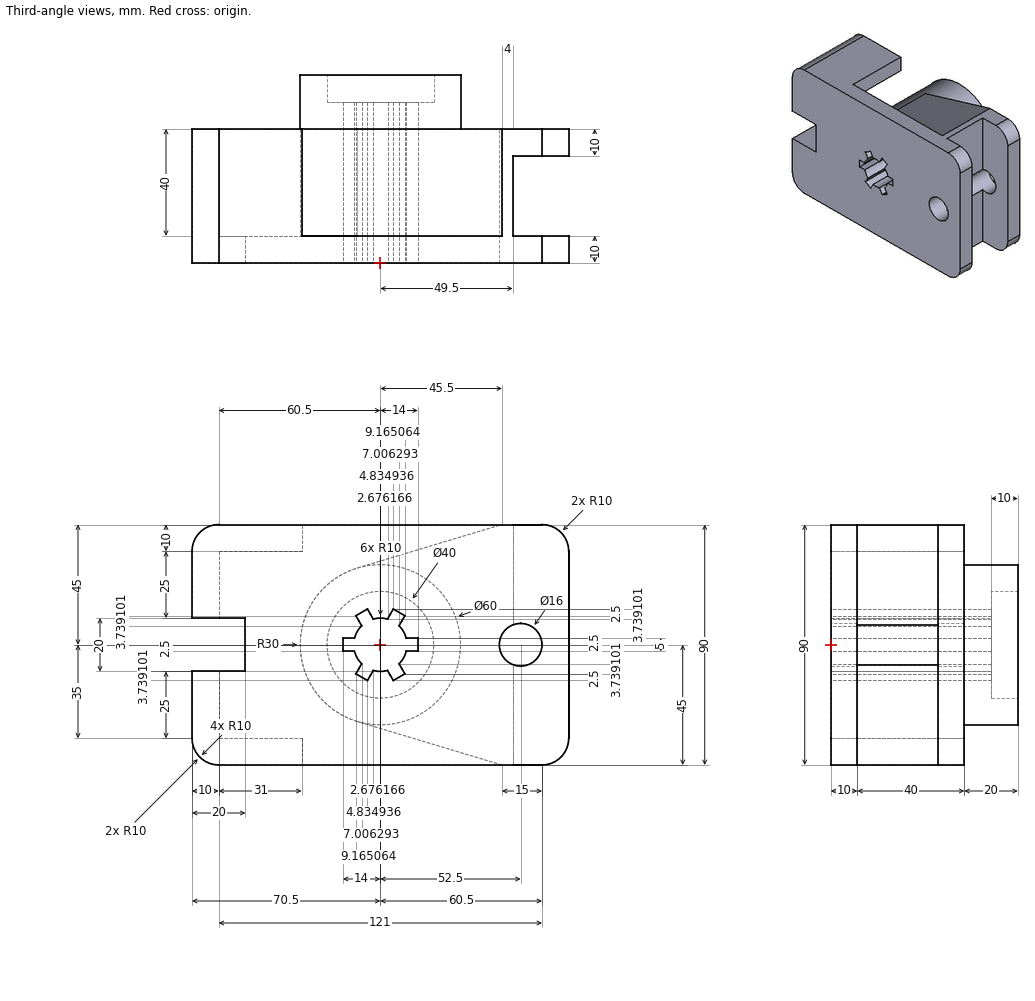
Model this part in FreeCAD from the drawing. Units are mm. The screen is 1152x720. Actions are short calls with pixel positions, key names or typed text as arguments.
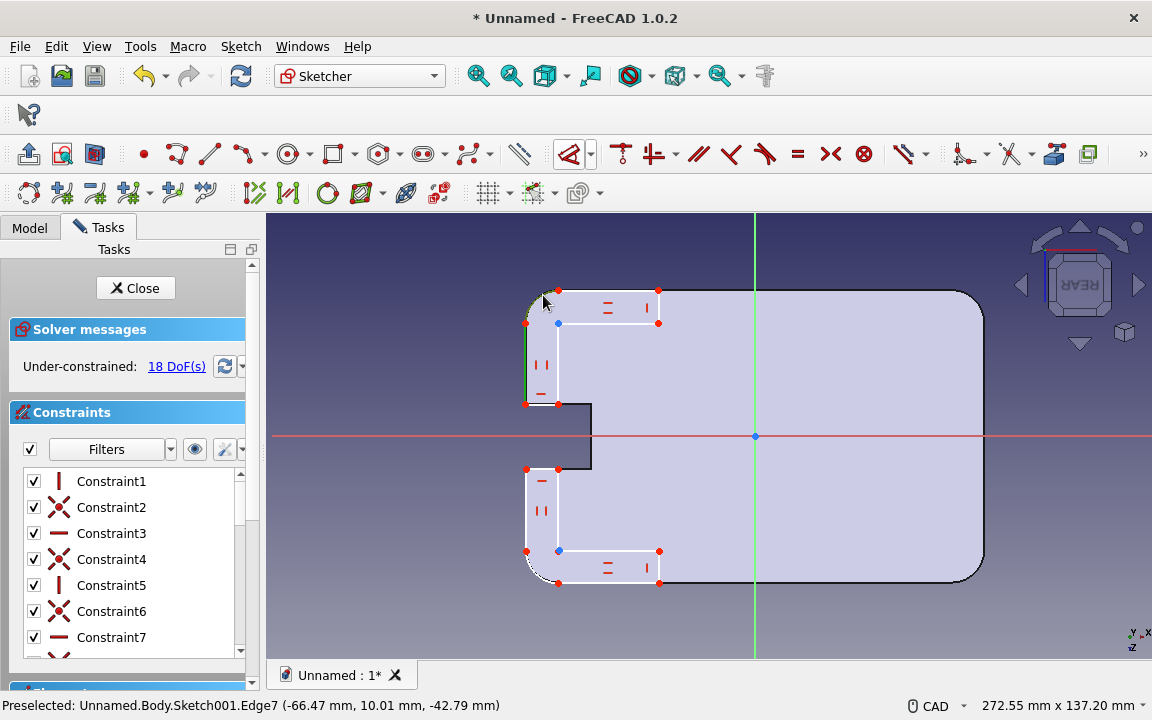
click(765, 154)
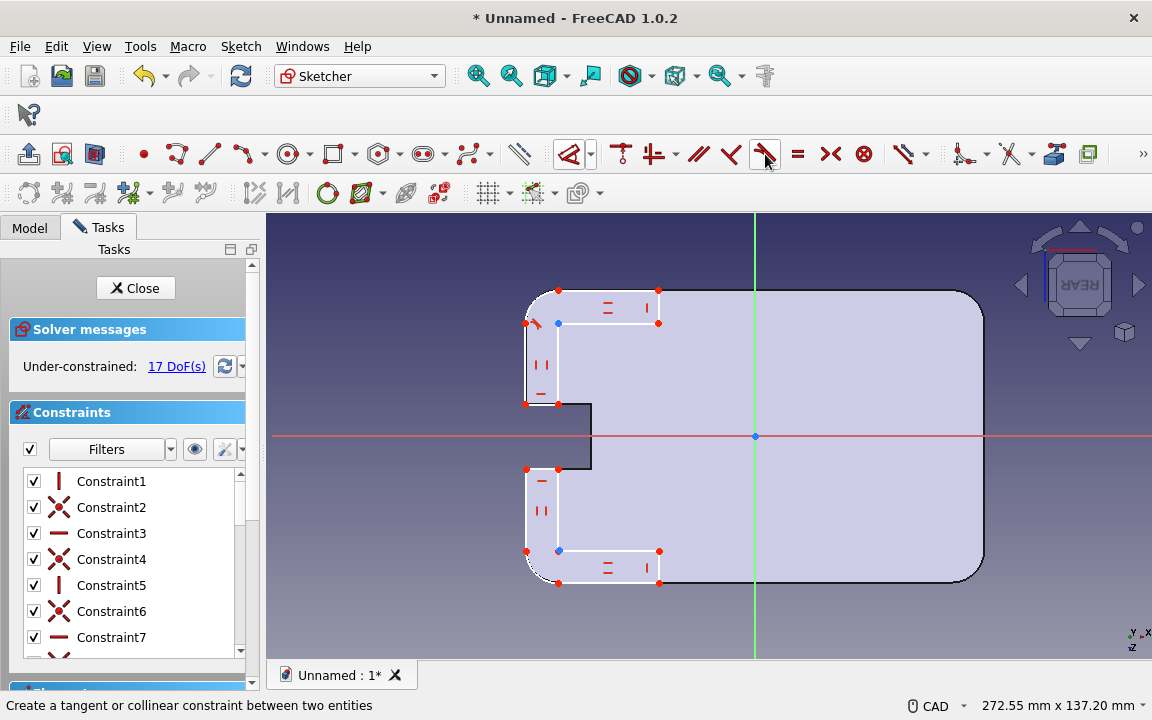
click(629, 291)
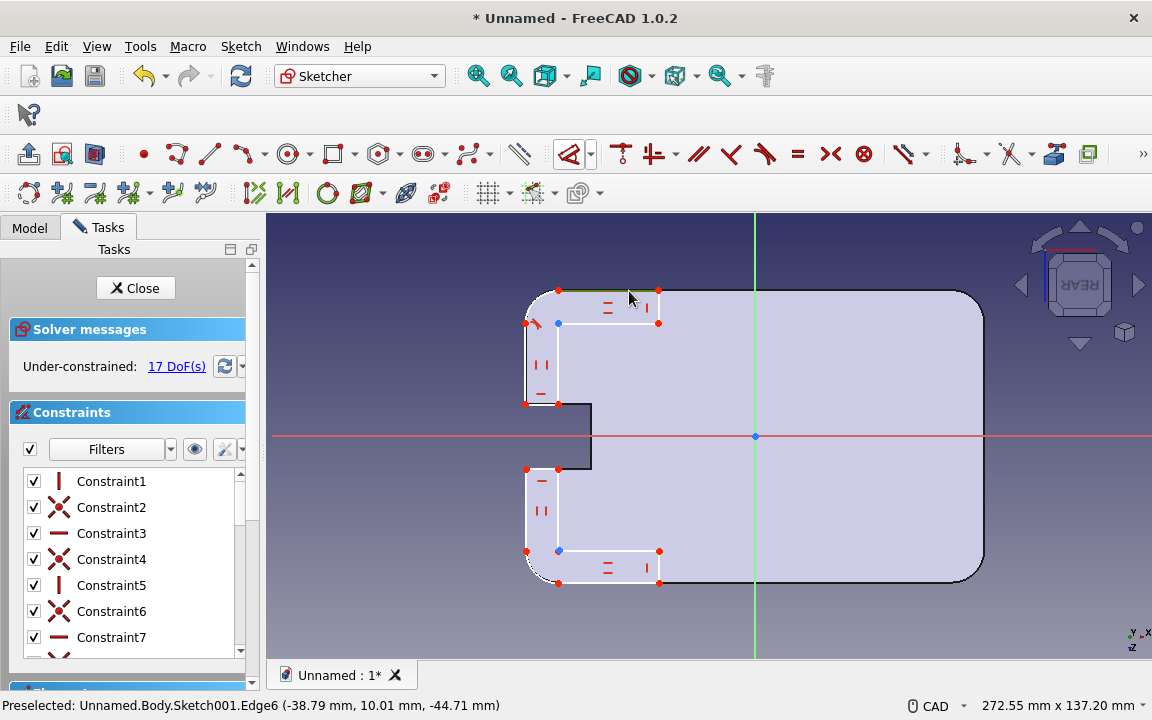
click(543, 295)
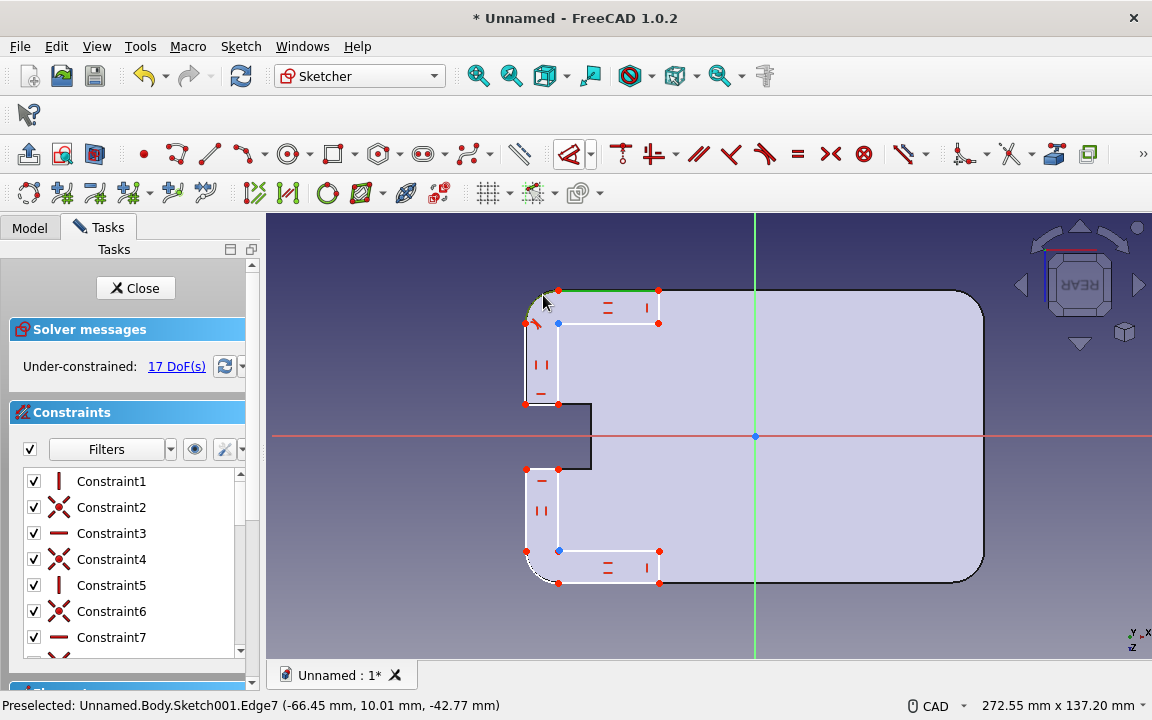
click(765, 154)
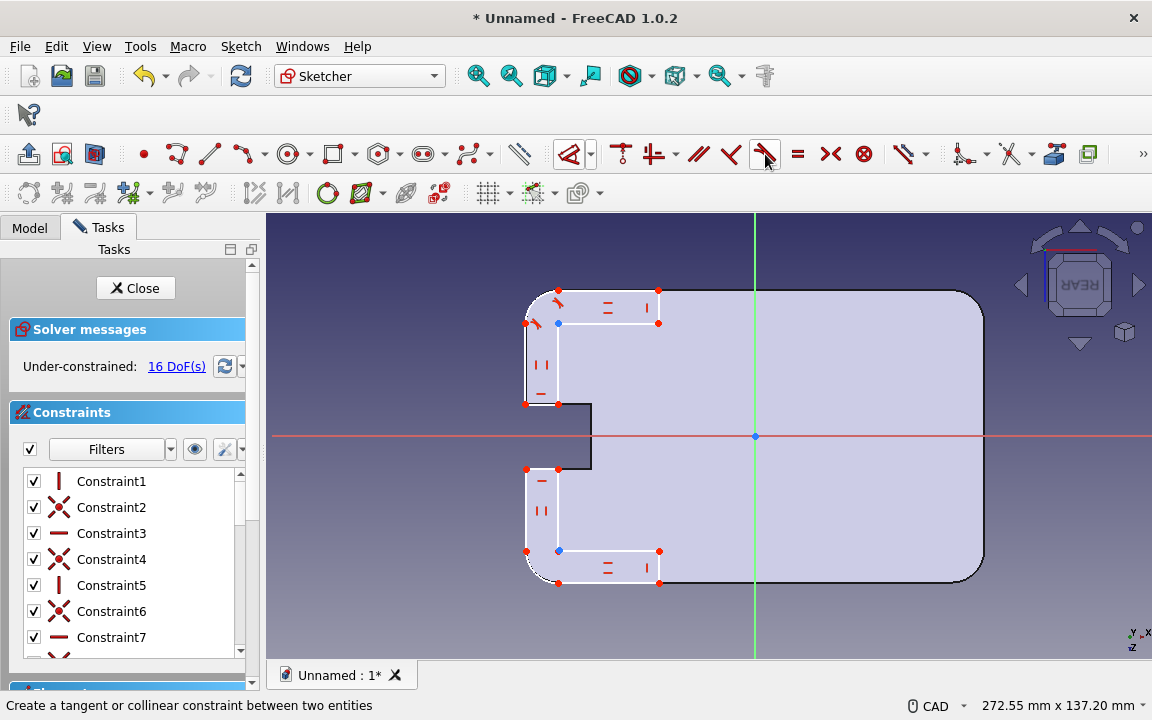
click(588, 583)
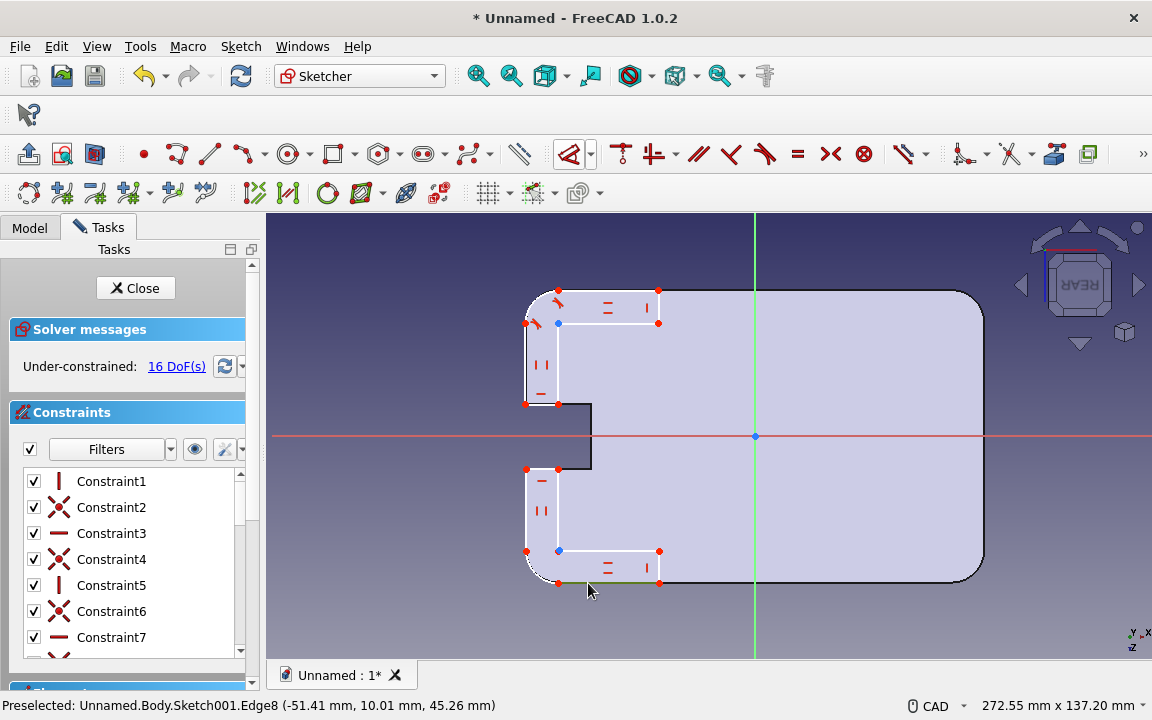
click(530, 566)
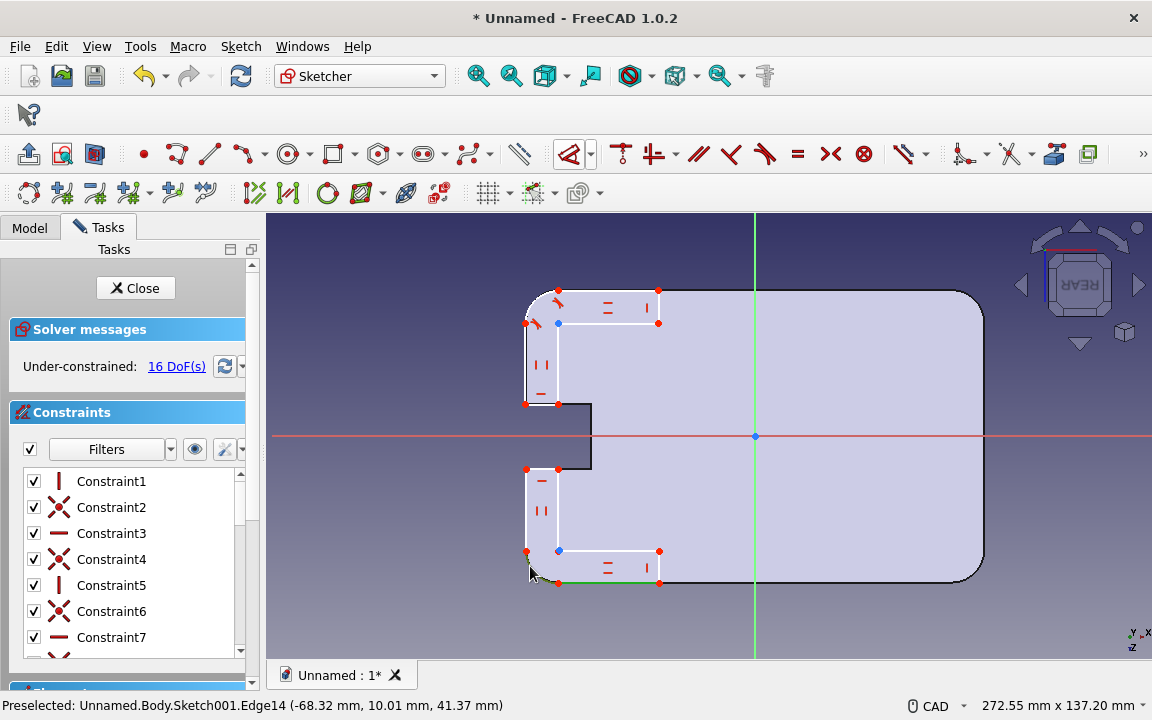
click(765, 154)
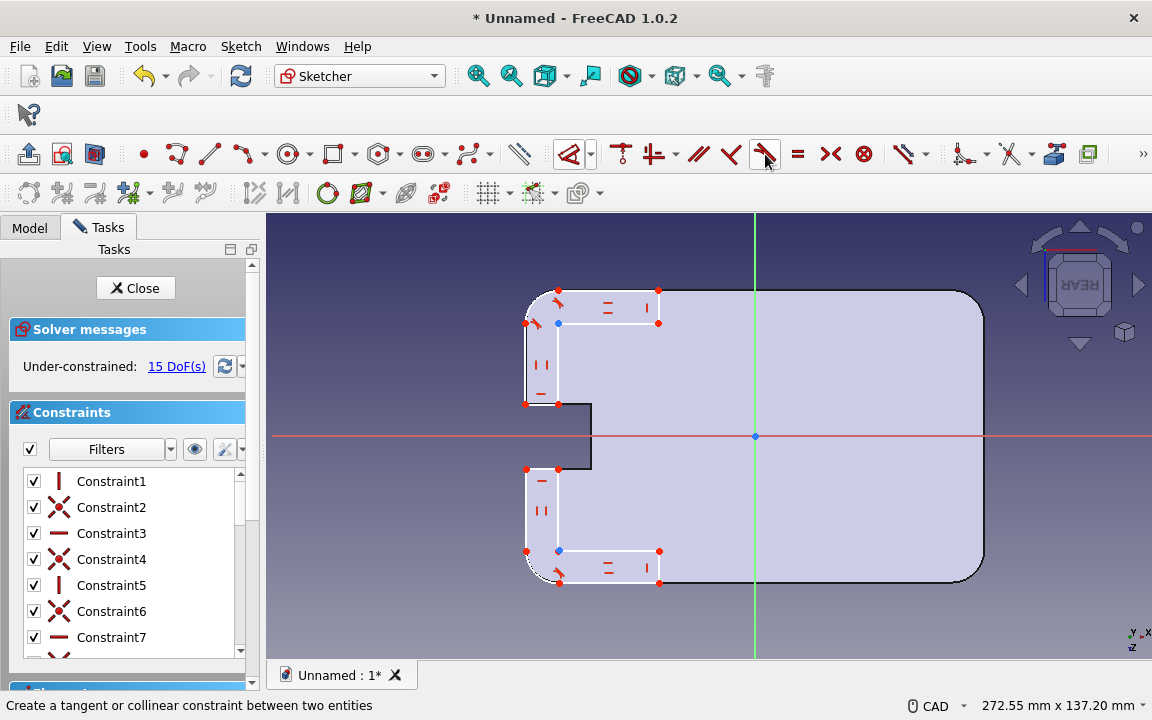
click(526, 494)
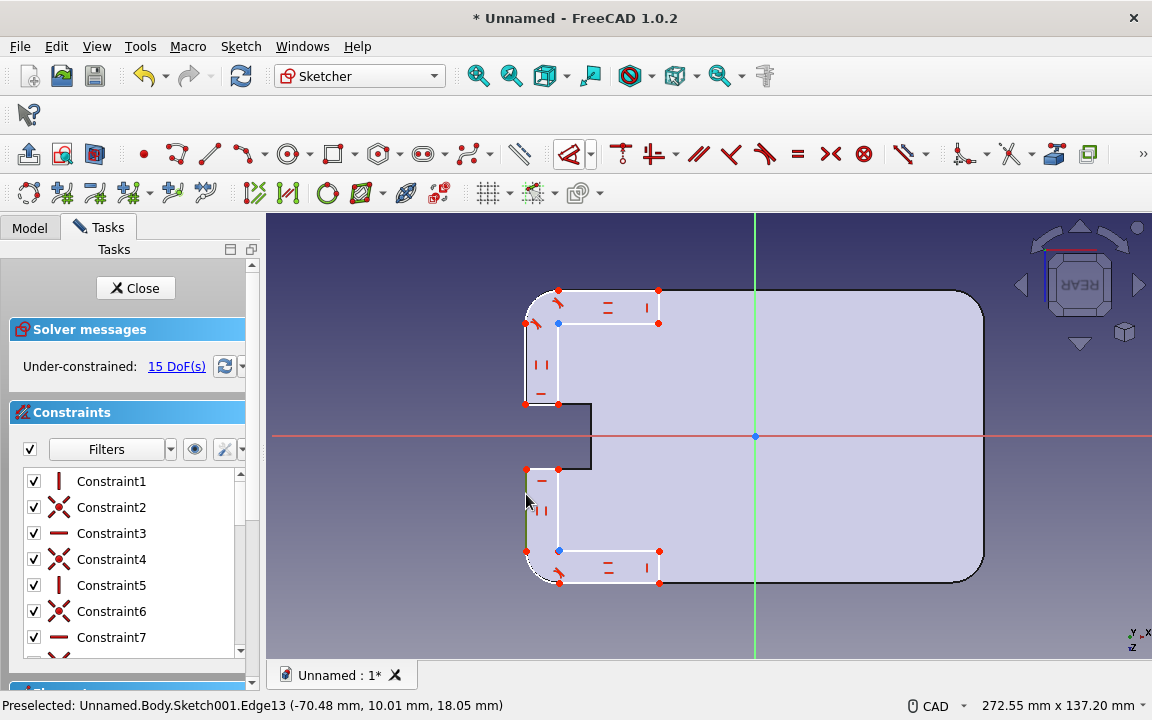
click(530, 566)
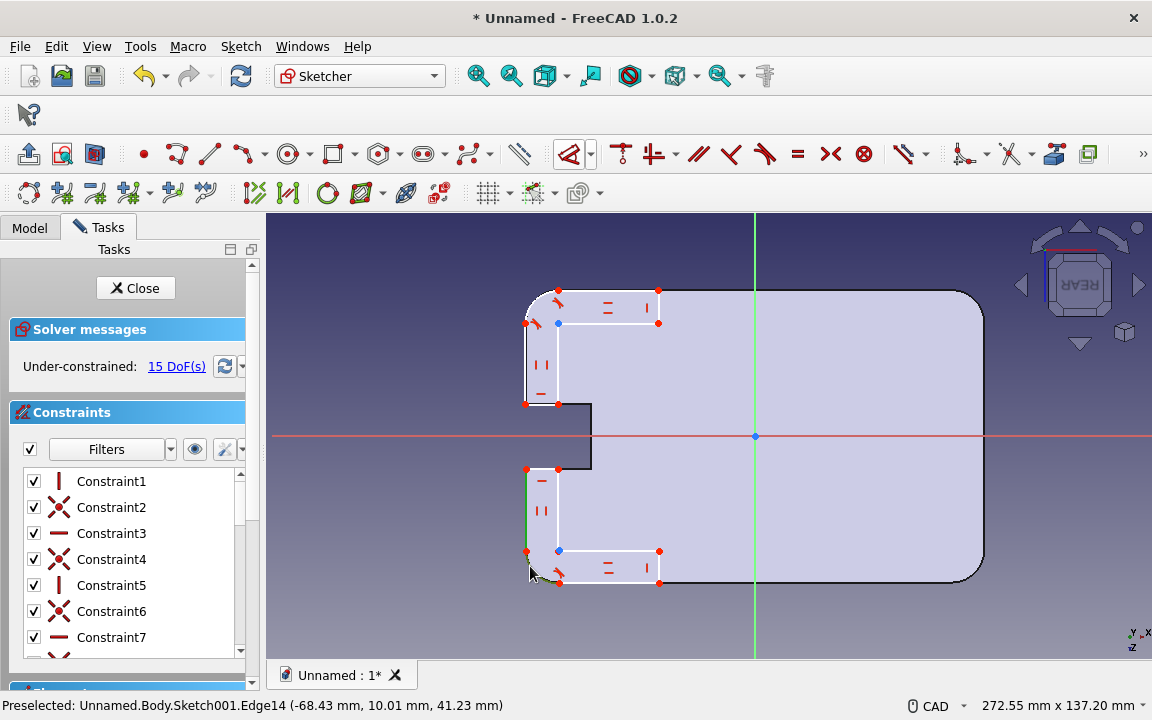
click(765, 154)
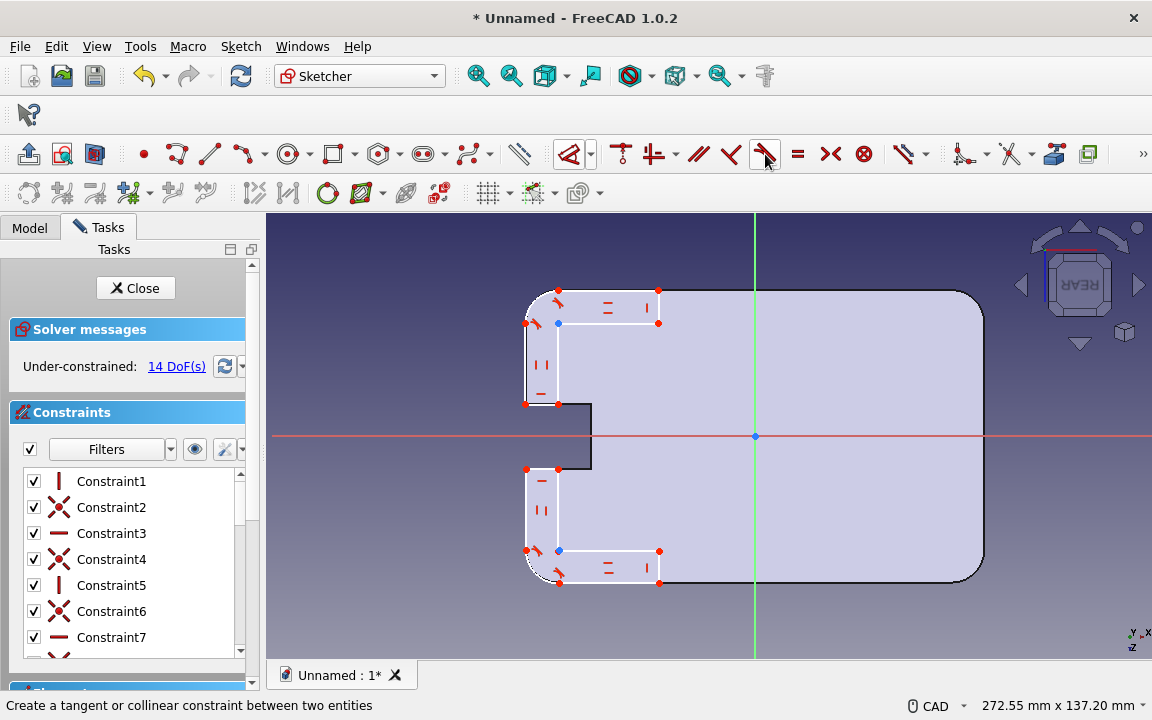
click(543, 295)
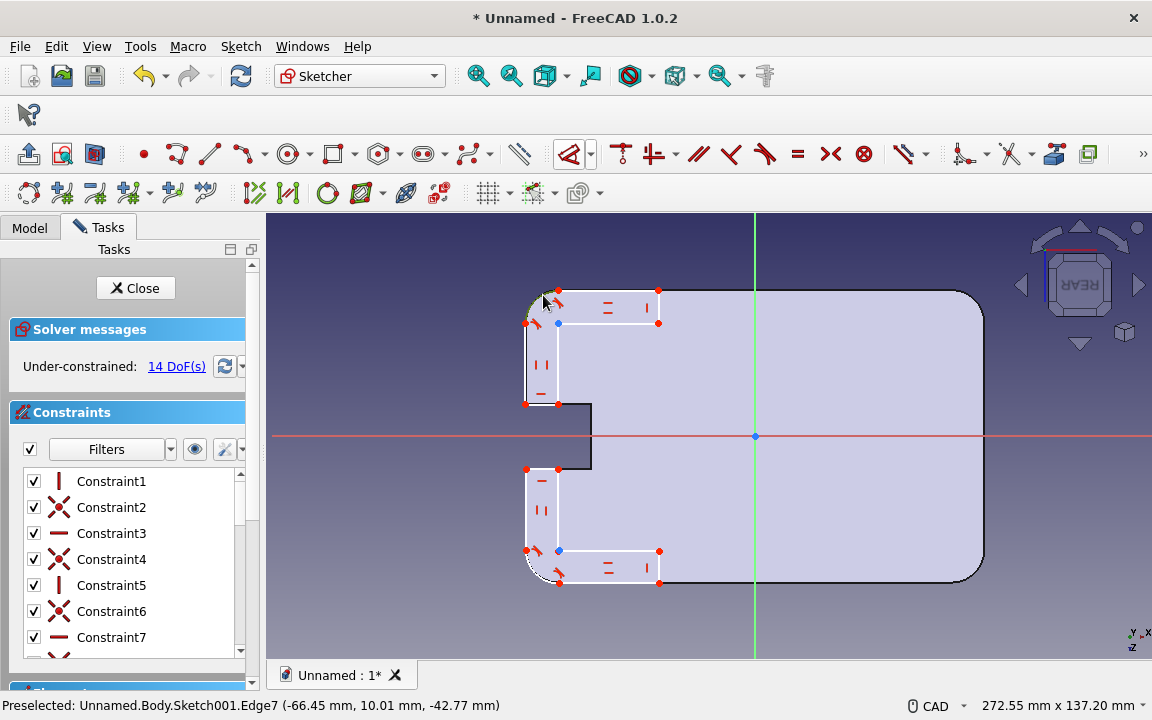
click(530, 565)